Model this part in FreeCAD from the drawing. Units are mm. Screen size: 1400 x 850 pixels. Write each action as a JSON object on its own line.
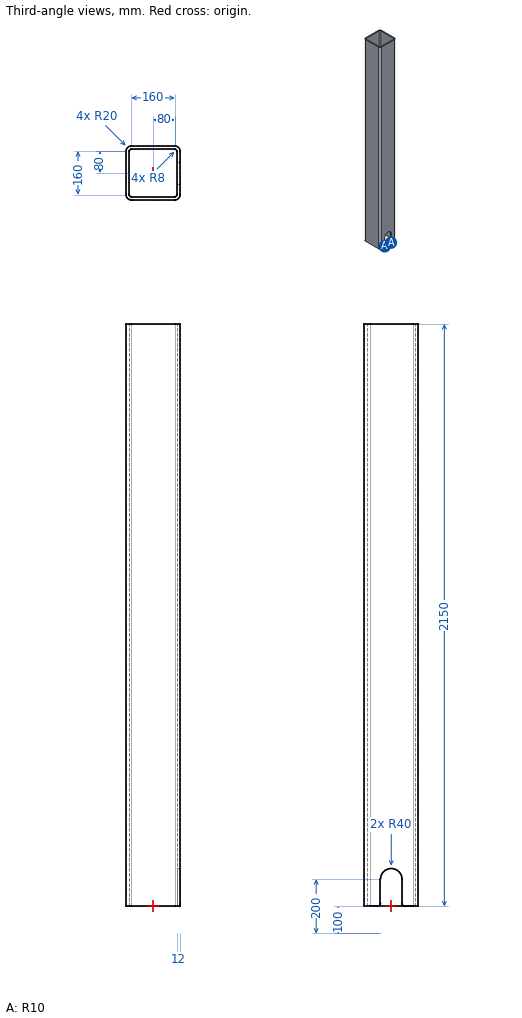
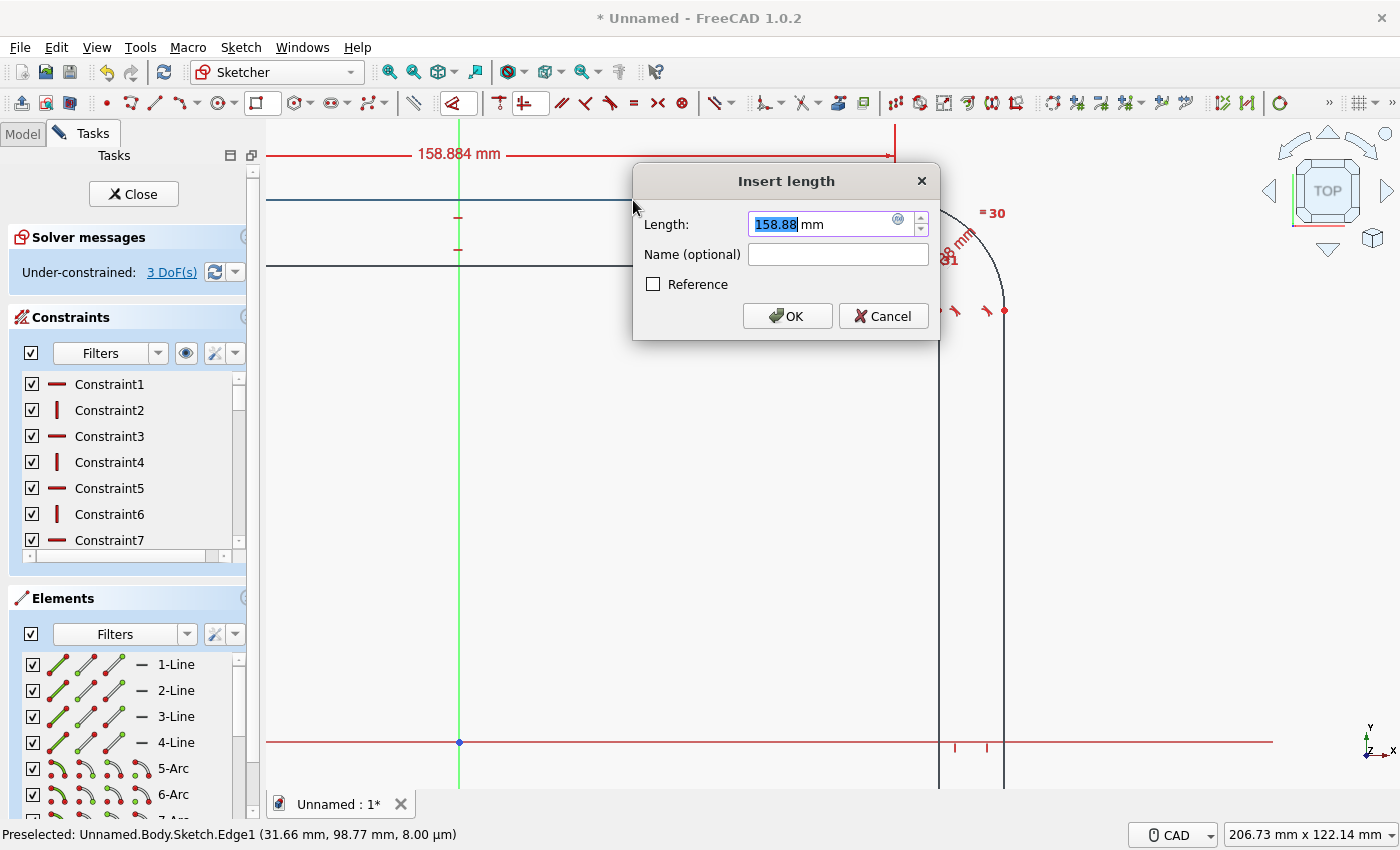
{"action": "type", "text": "160"}
{"action": "key", "text": "Return"}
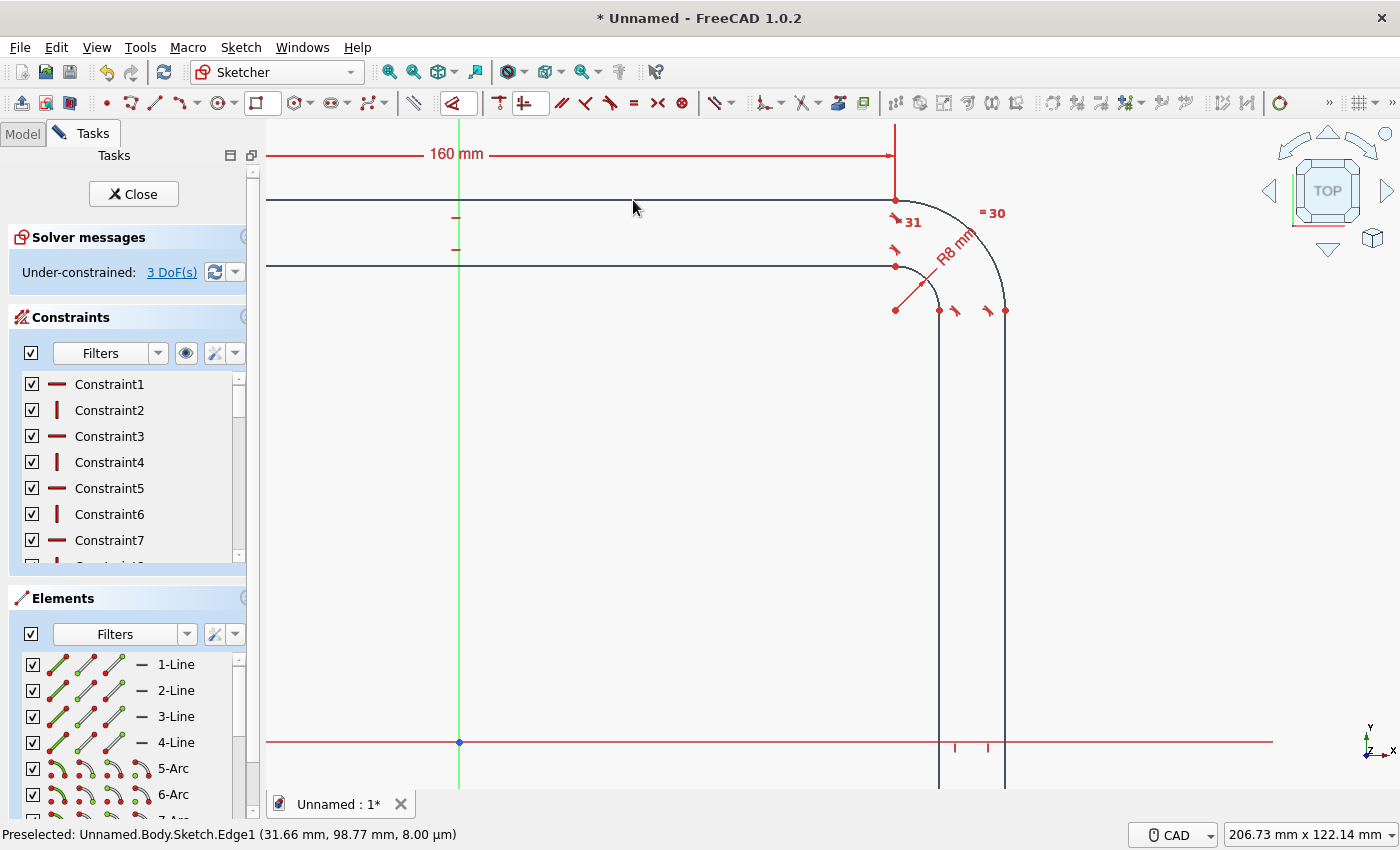
{"action": "scroll", "coordinate": [942, 286], "scroll_direction": "down", "scroll_amount": 5}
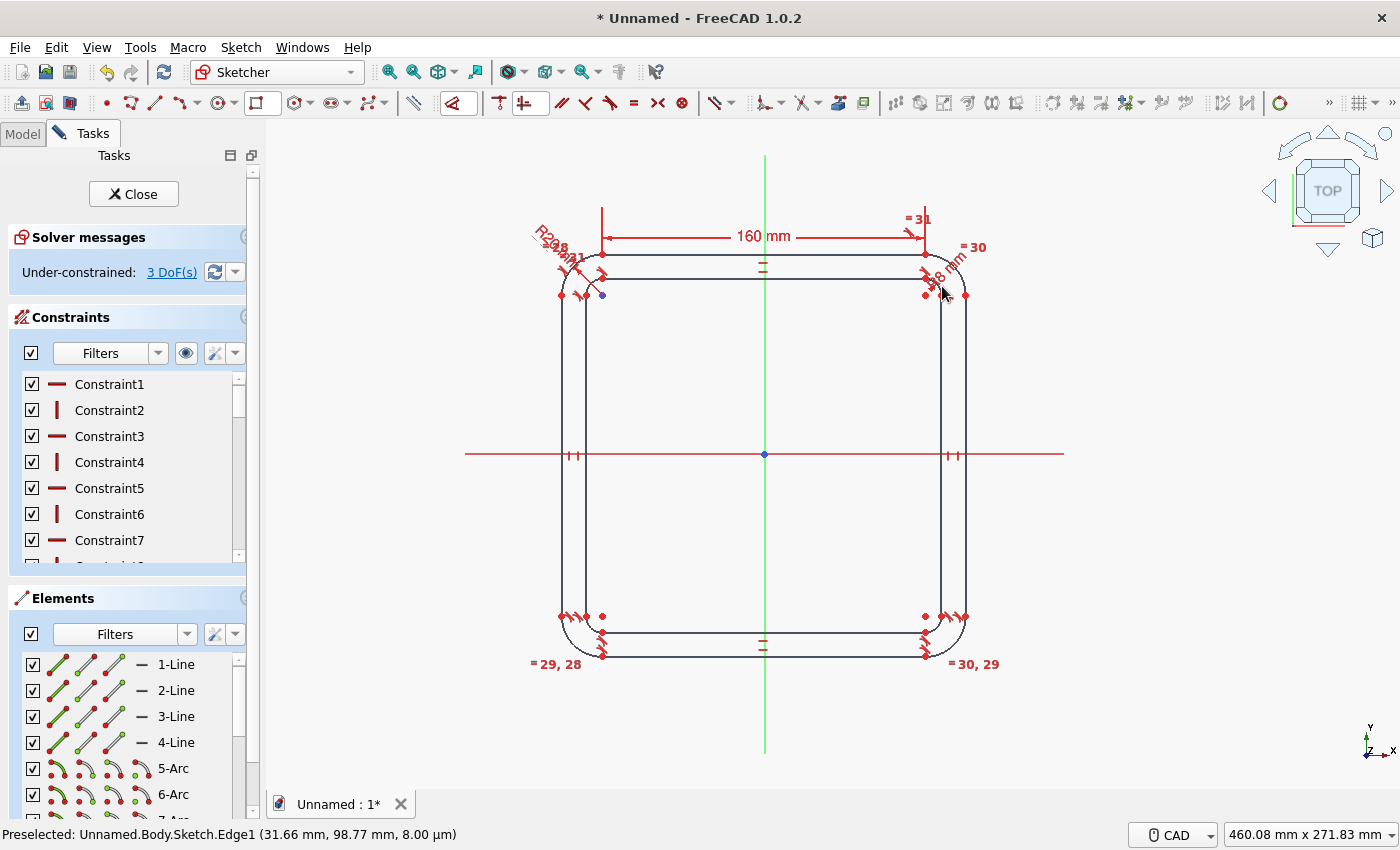
{"action": "left_click", "coordinate": [562, 392]}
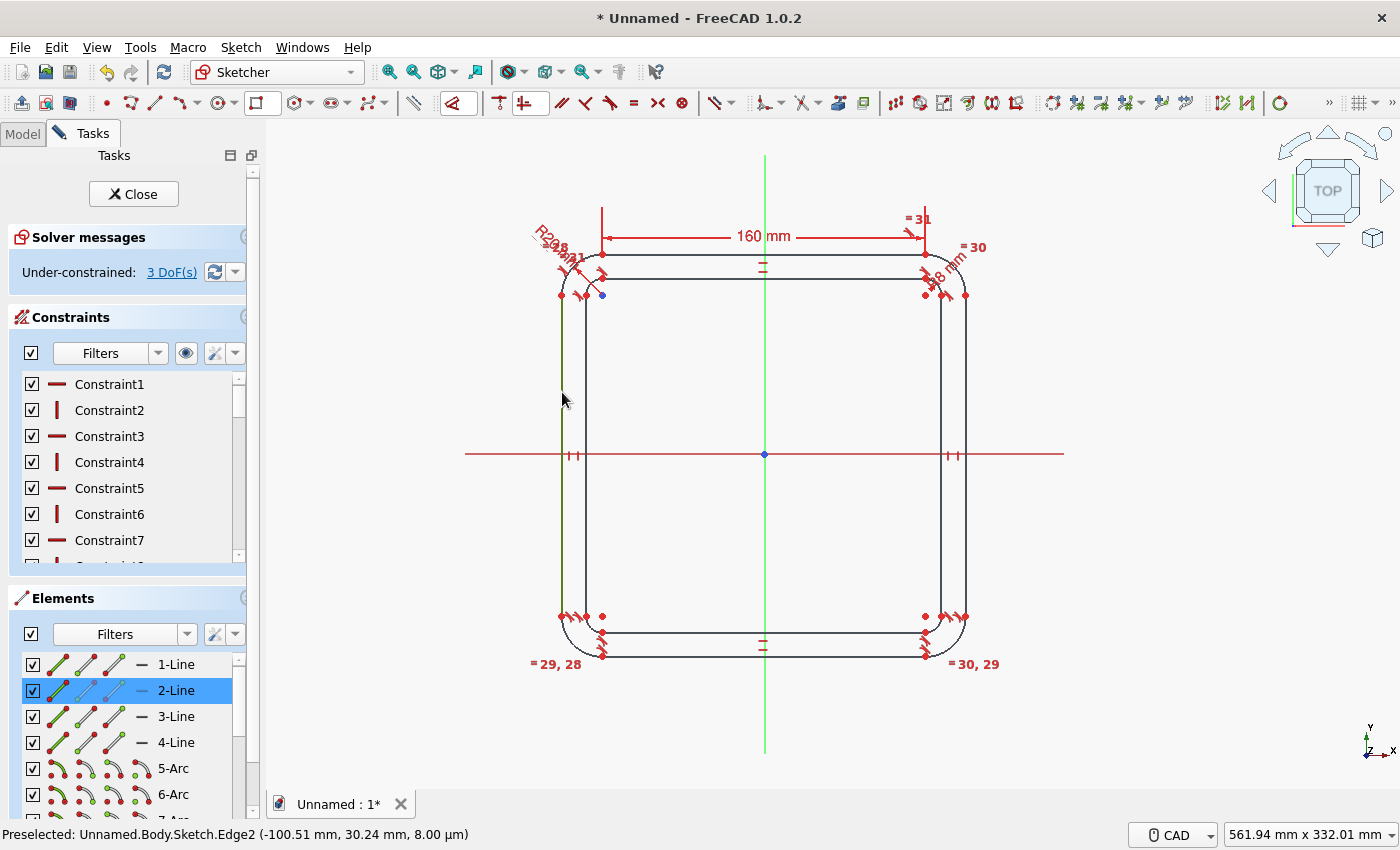
{"action": "left_click", "coordinate": [472, 104]}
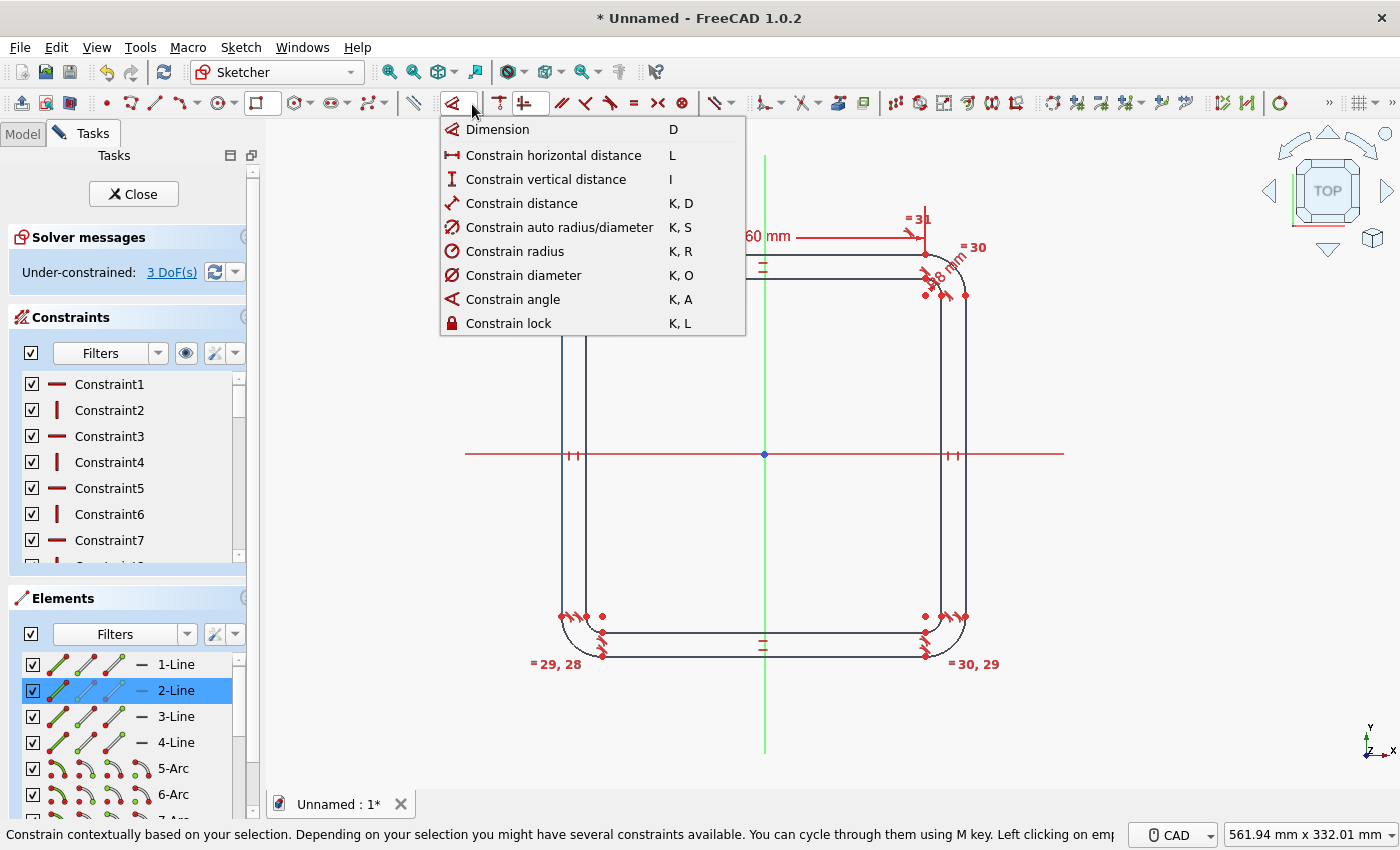
{"action": "left_click", "coordinate": [593, 179]}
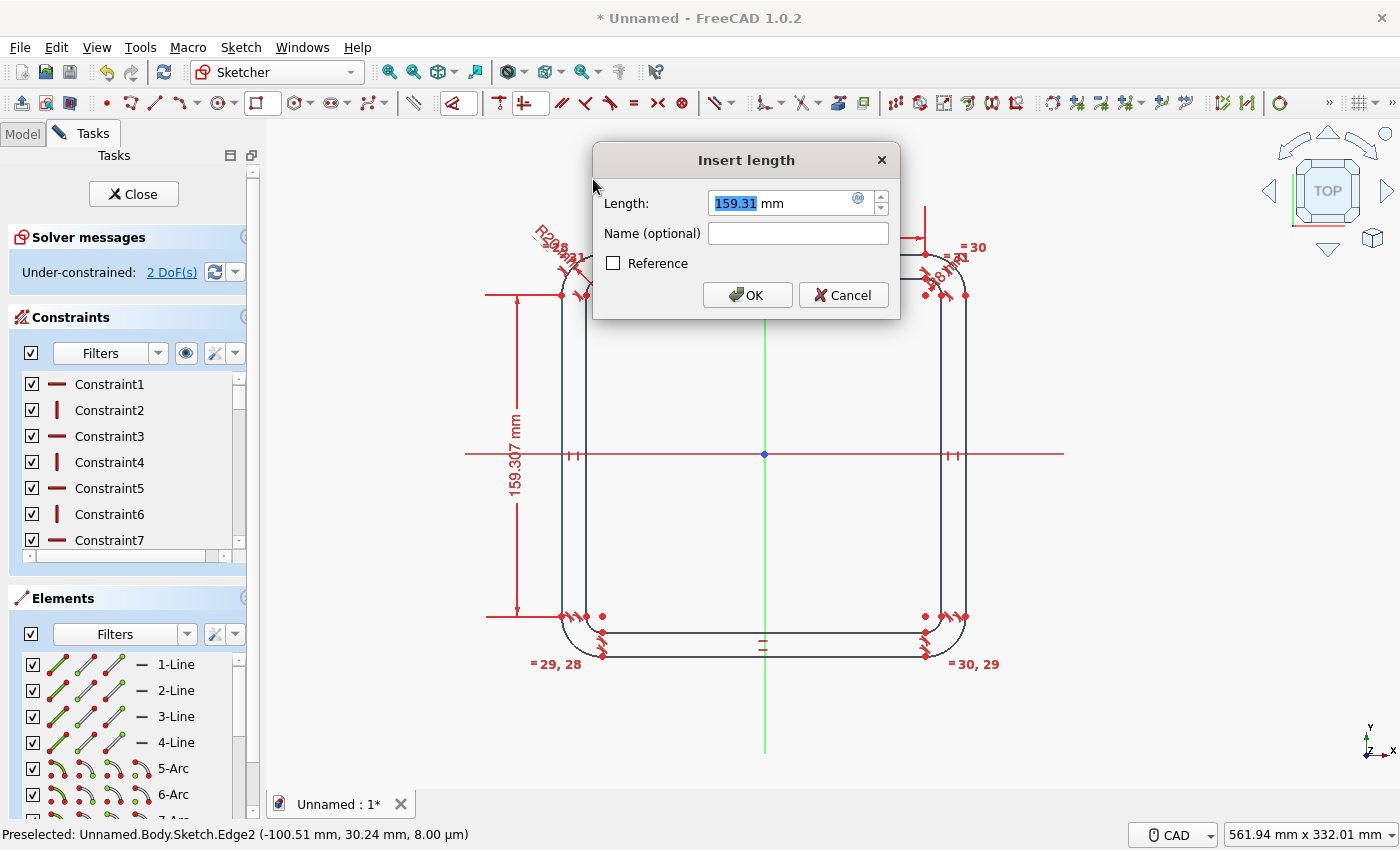
{"action": "type", "text": "160"}
{"action": "key", "text": "Return"}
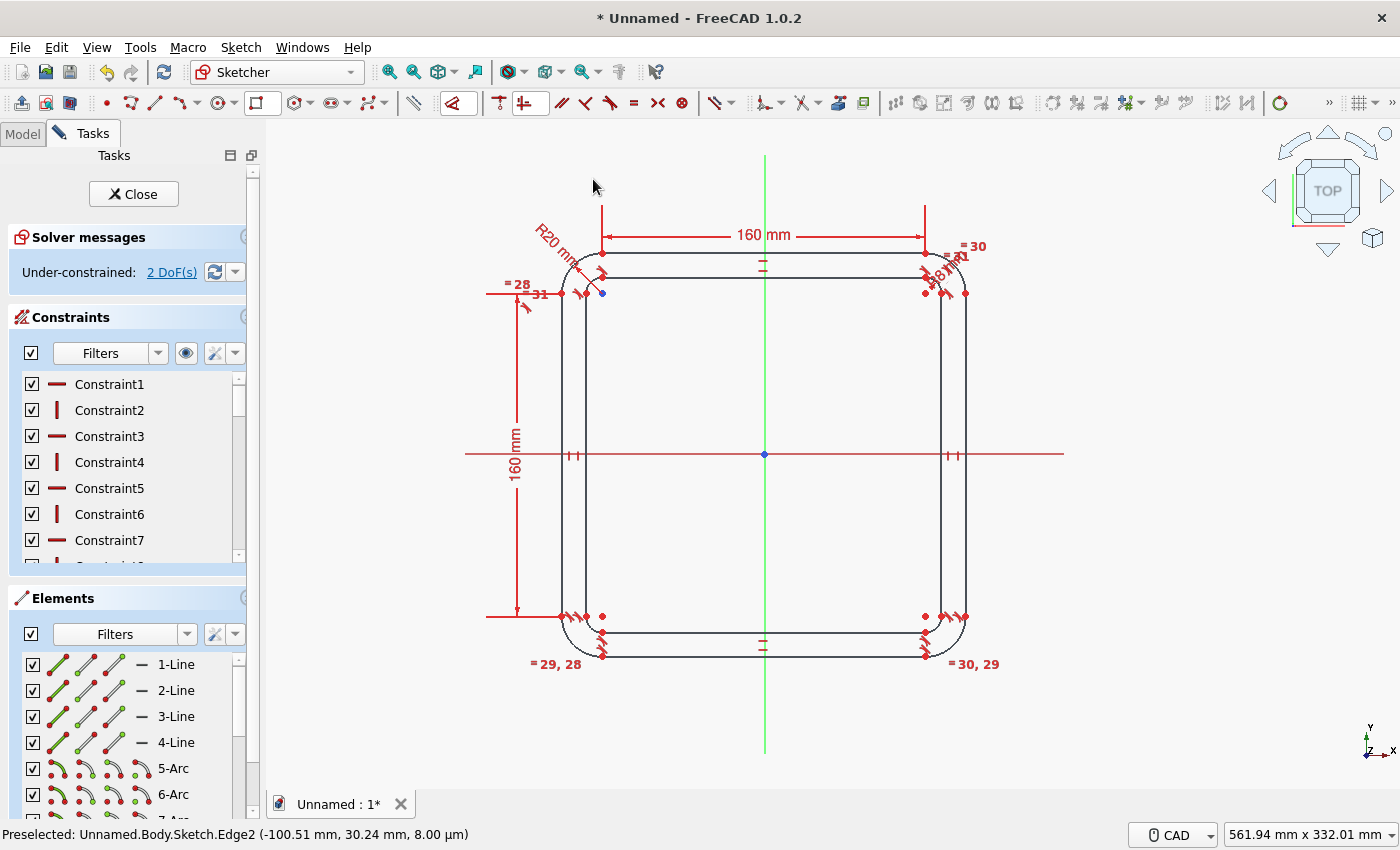
{"action": "left_click", "coordinate": [925, 253]}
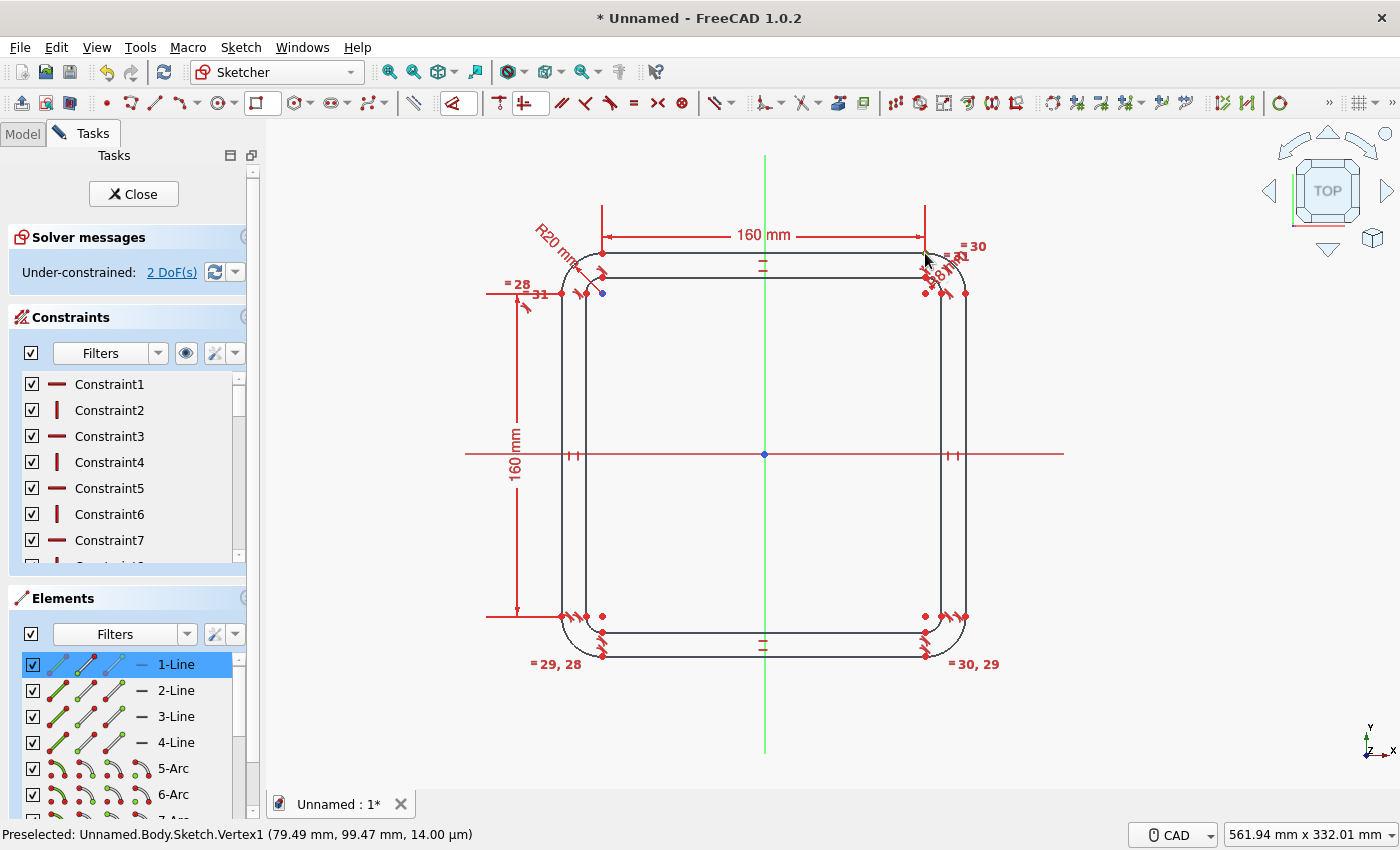
{"action": "left_click", "coordinate": [472, 104]}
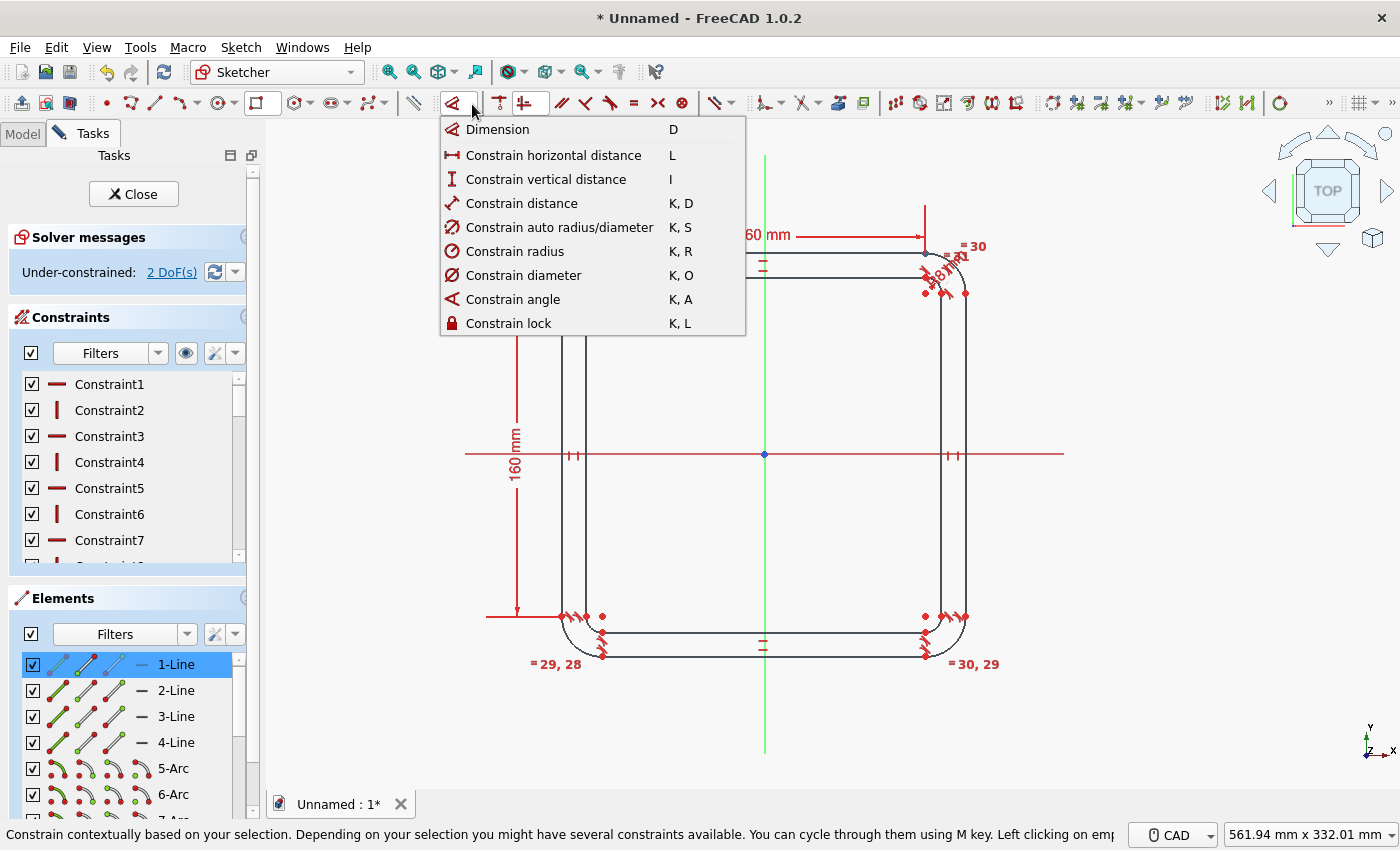
{"action": "left_click", "coordinate": [593, 155]}